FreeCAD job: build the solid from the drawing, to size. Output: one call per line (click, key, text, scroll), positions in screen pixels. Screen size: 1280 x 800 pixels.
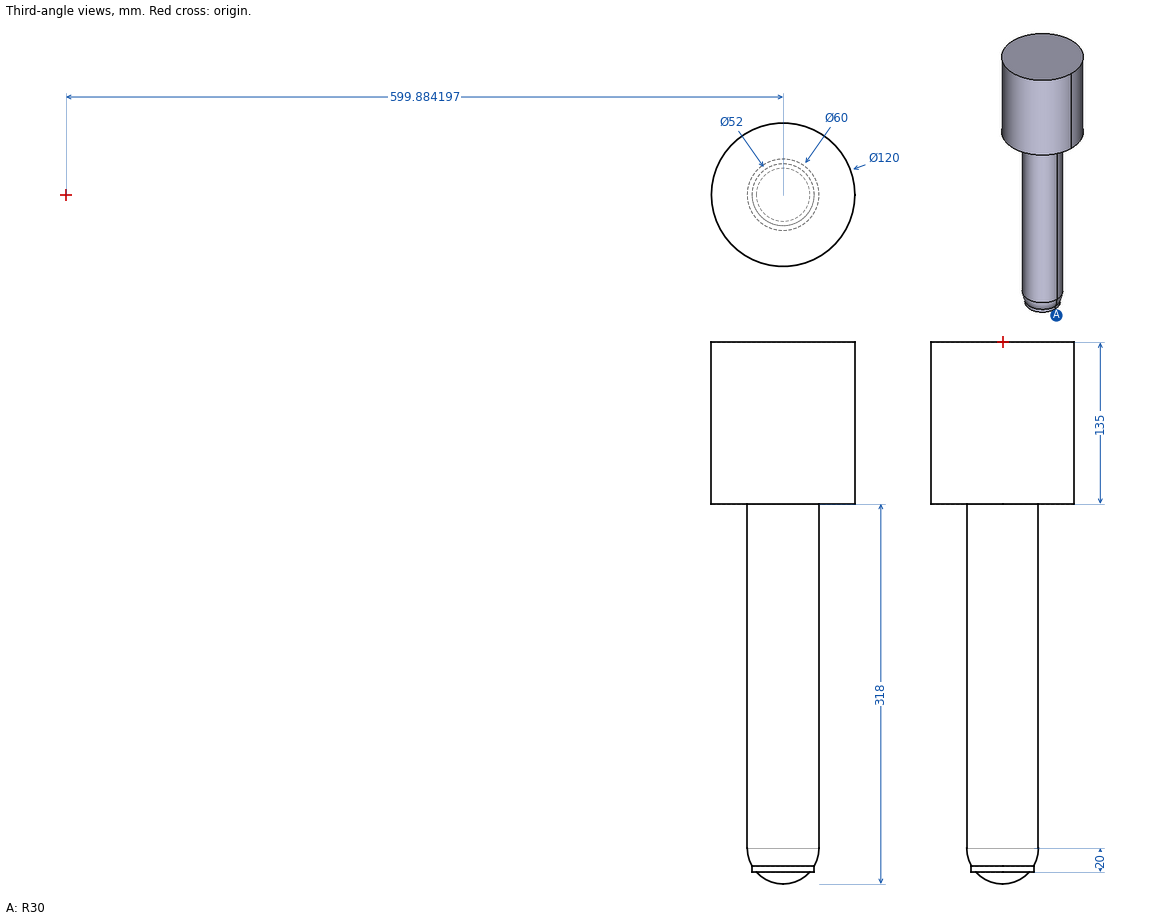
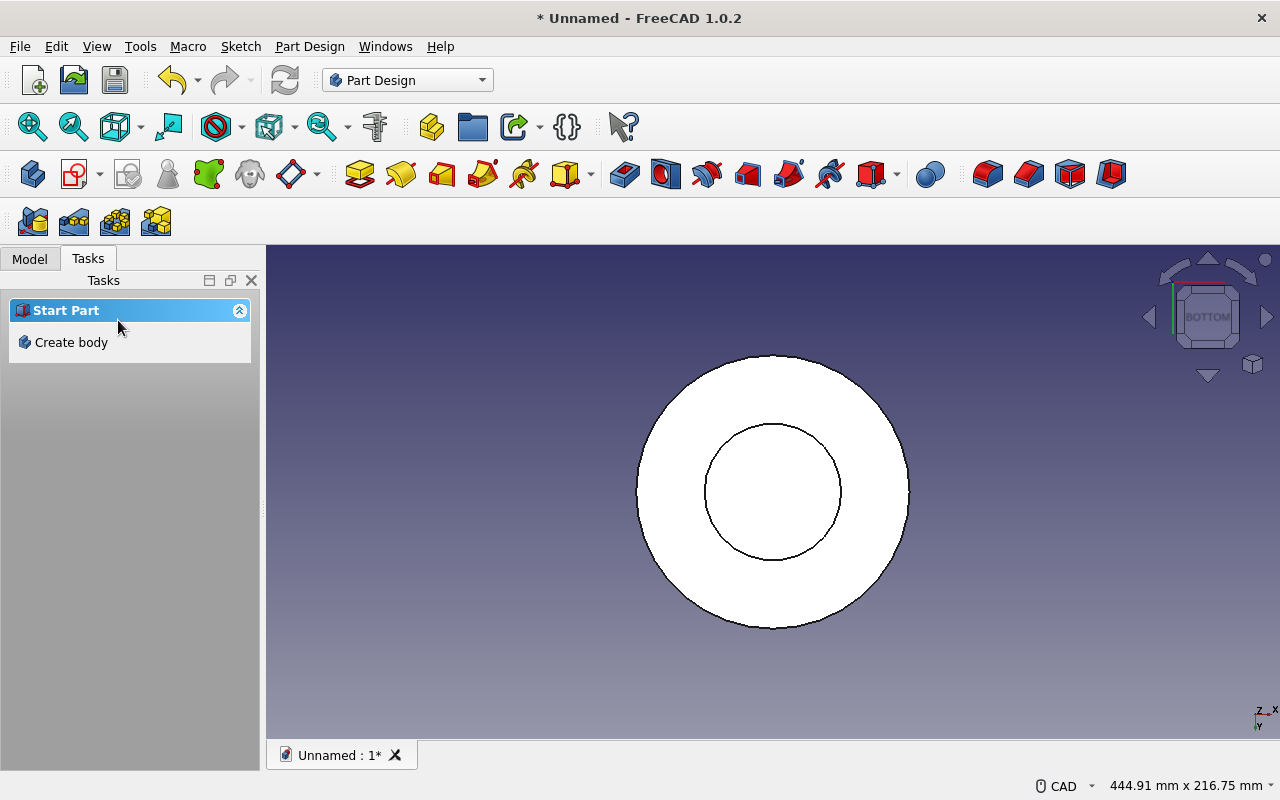
click(704, 491)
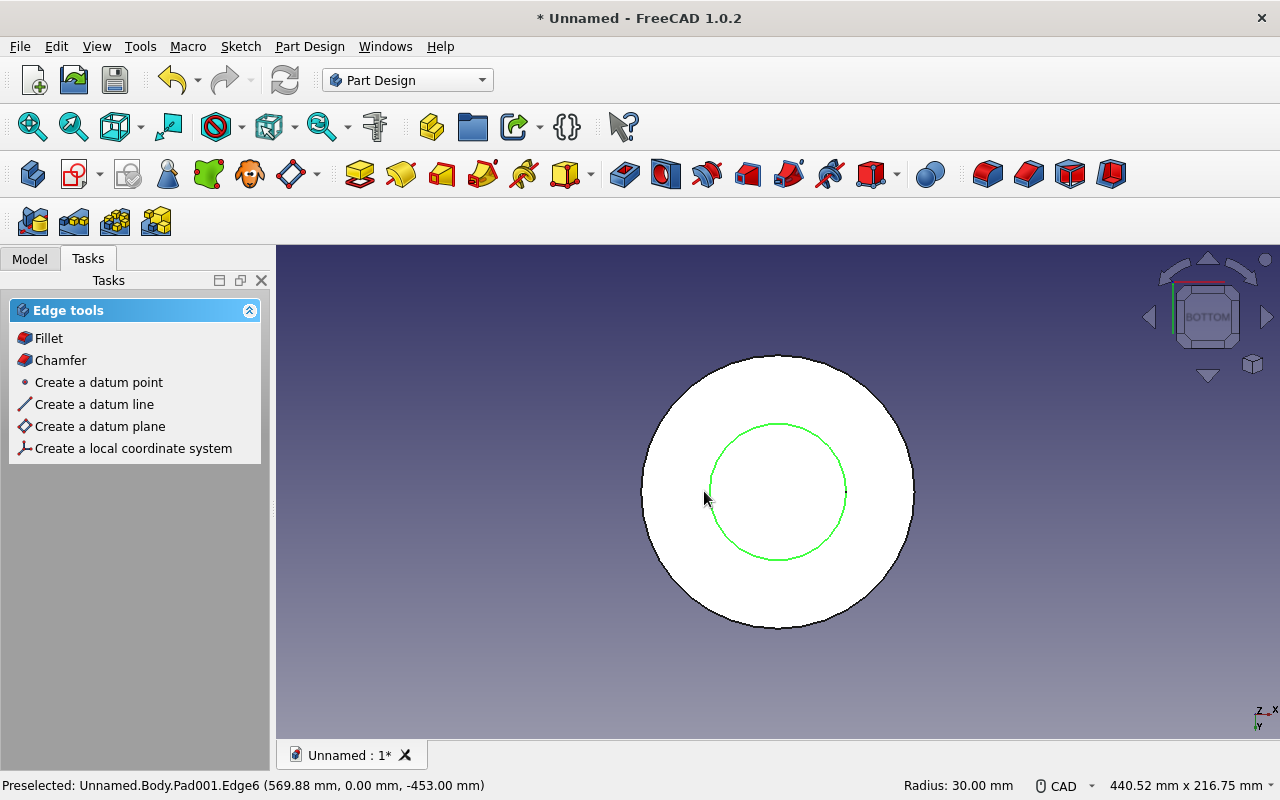
click(988, 174)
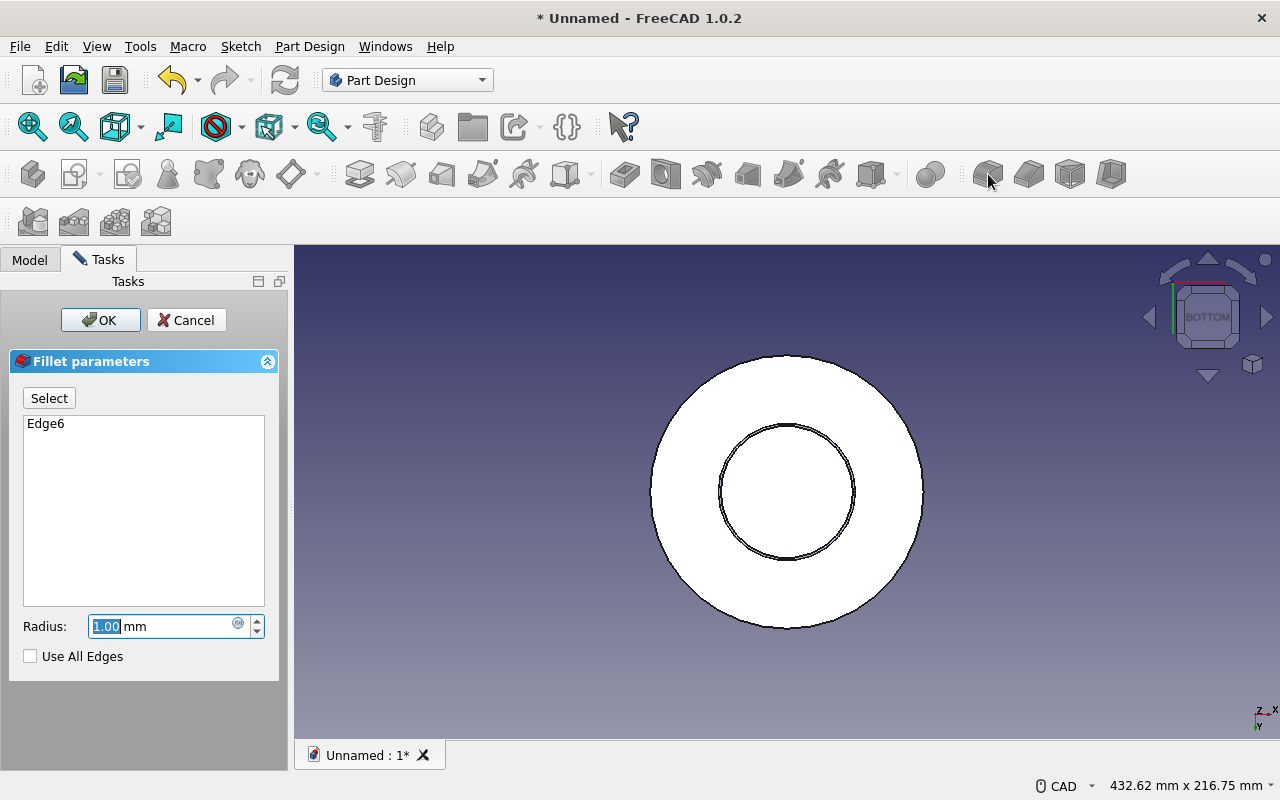
text(30)
key(Tab)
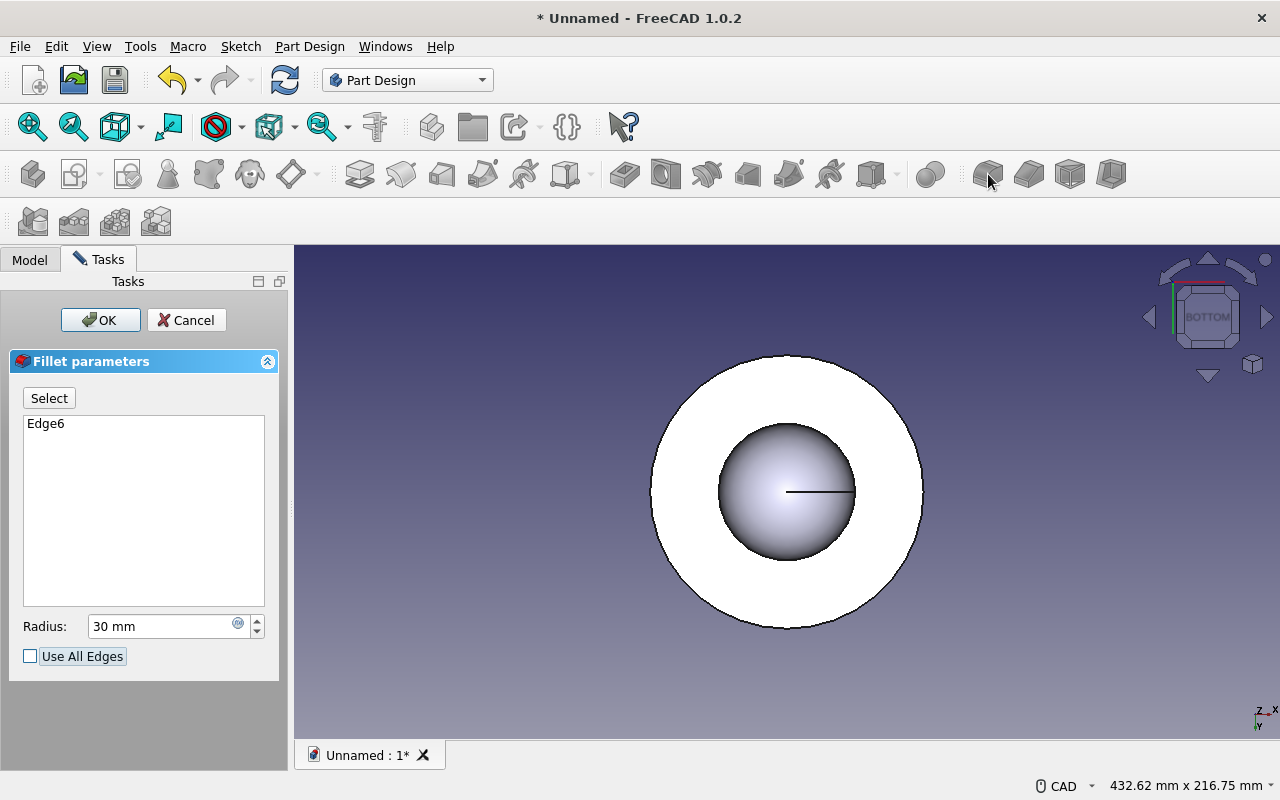
click(101, 320)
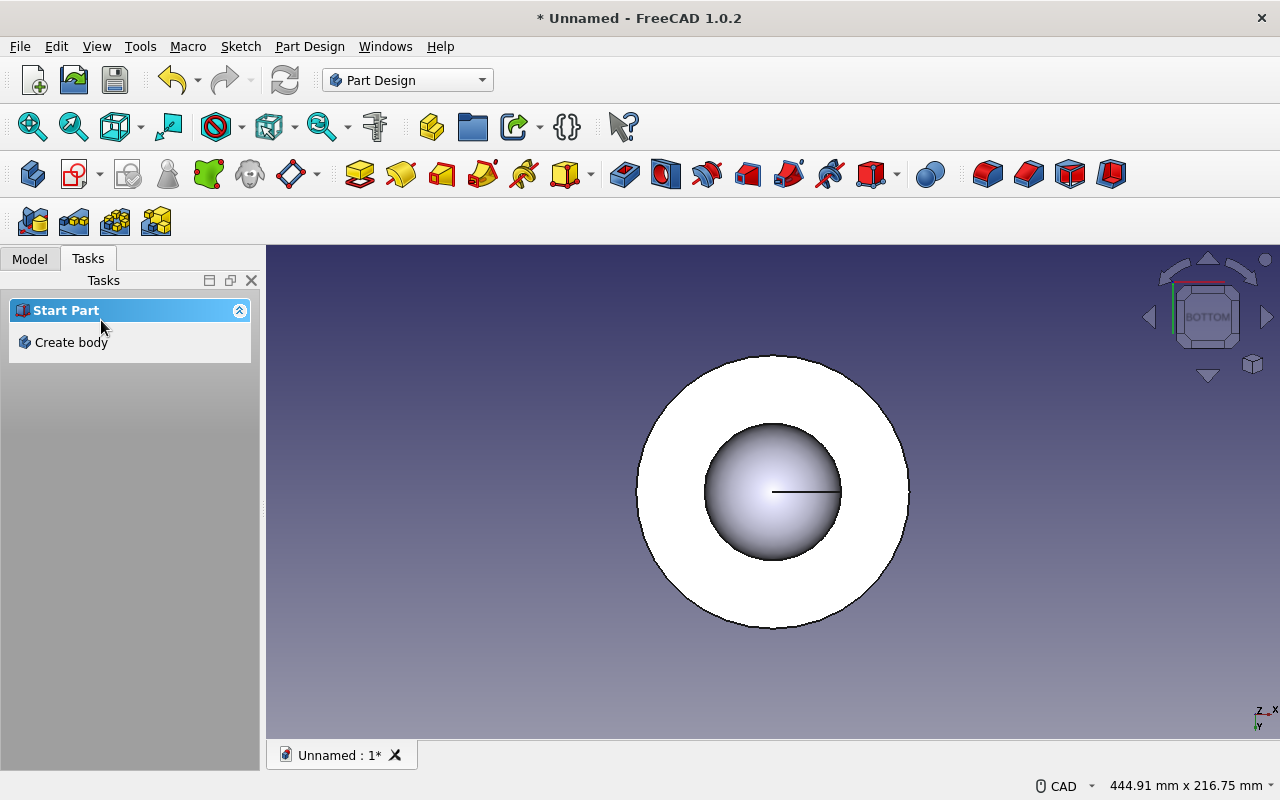
click(30, 258)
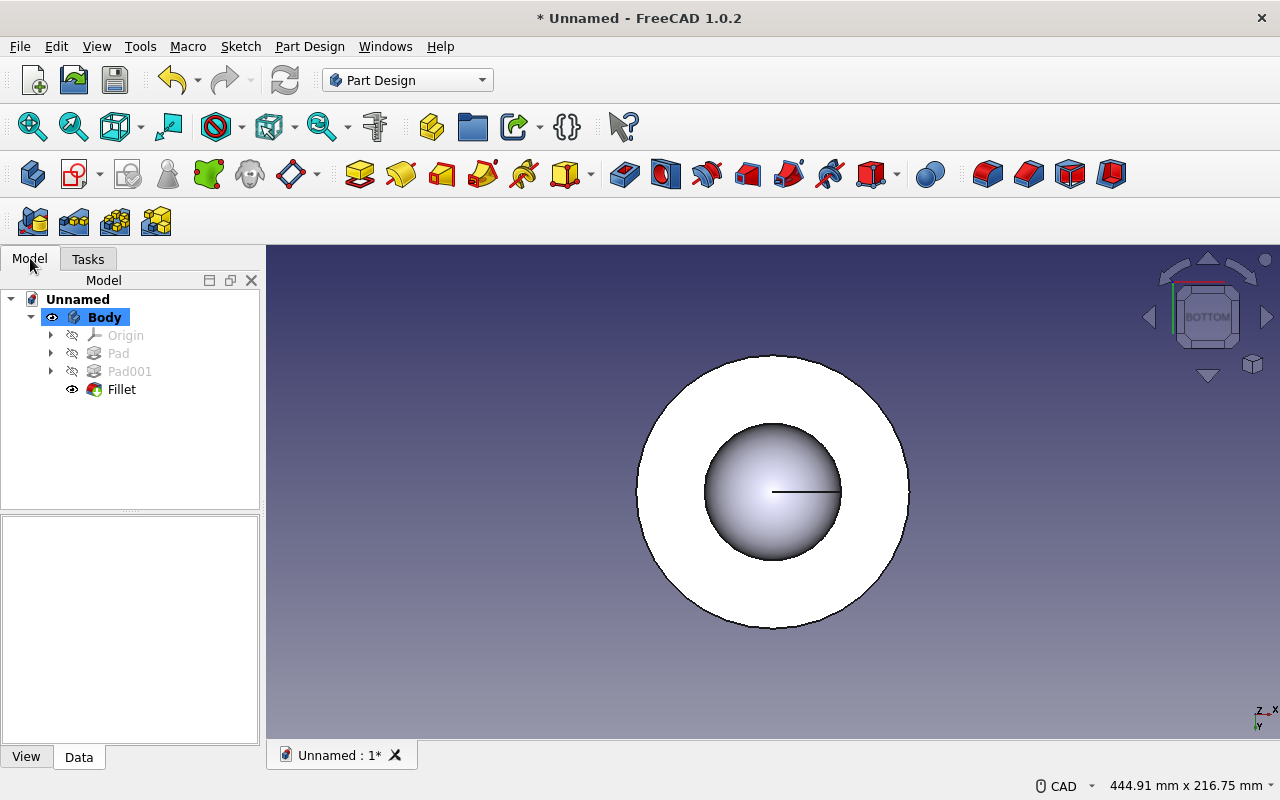
click(51, 335)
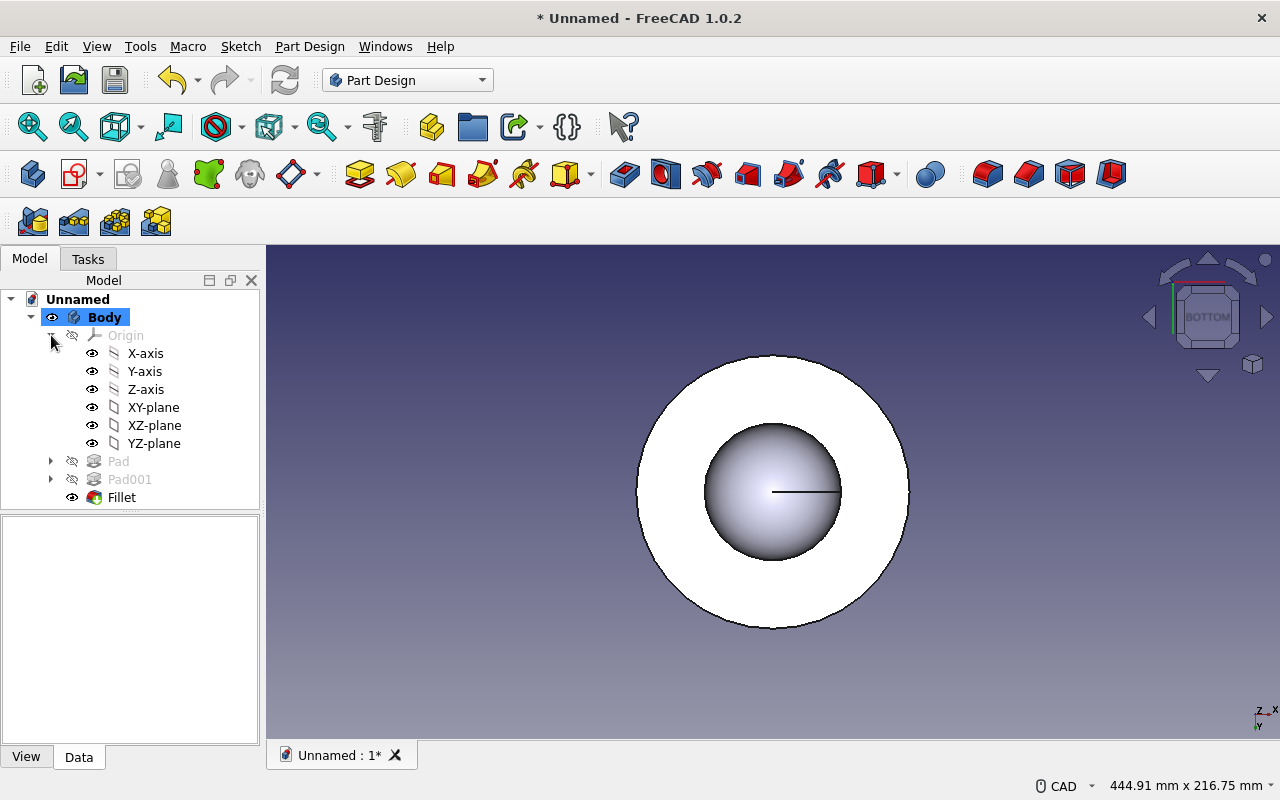
click(137, 407)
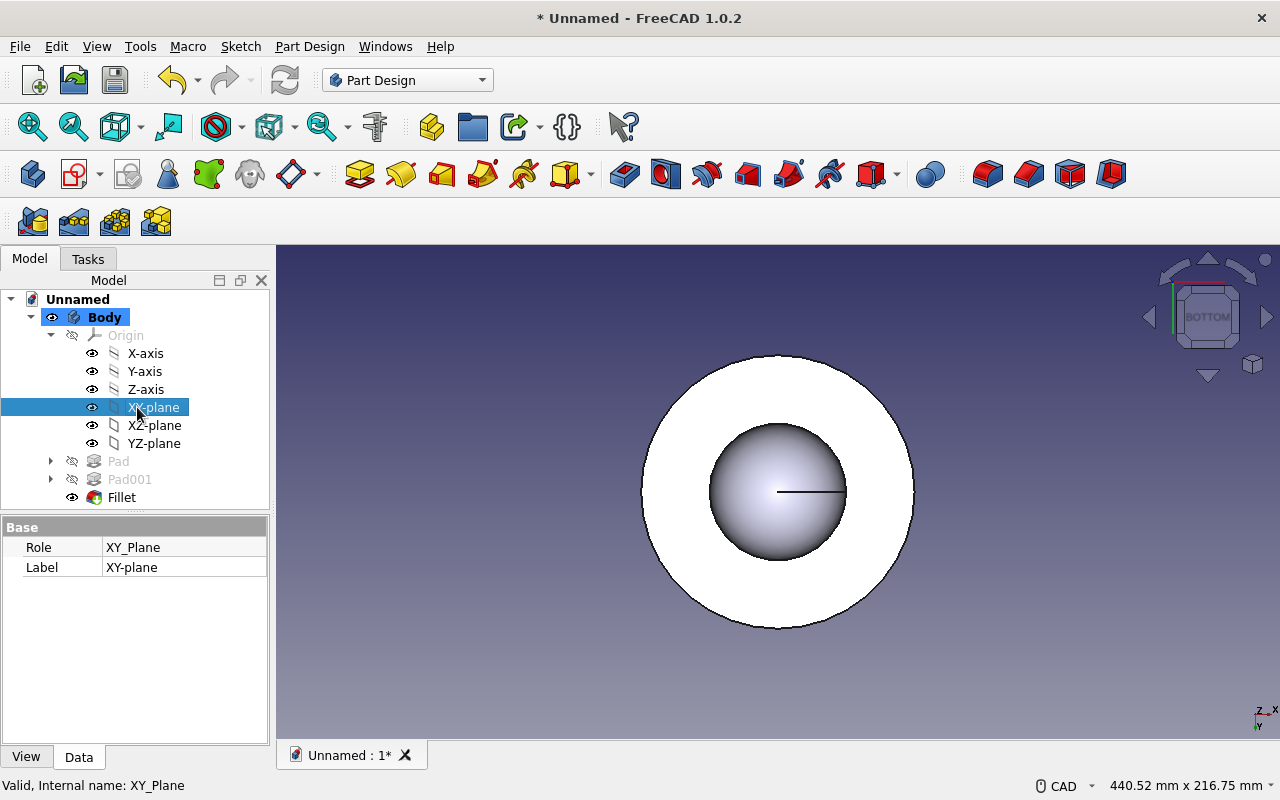
click(290, 174)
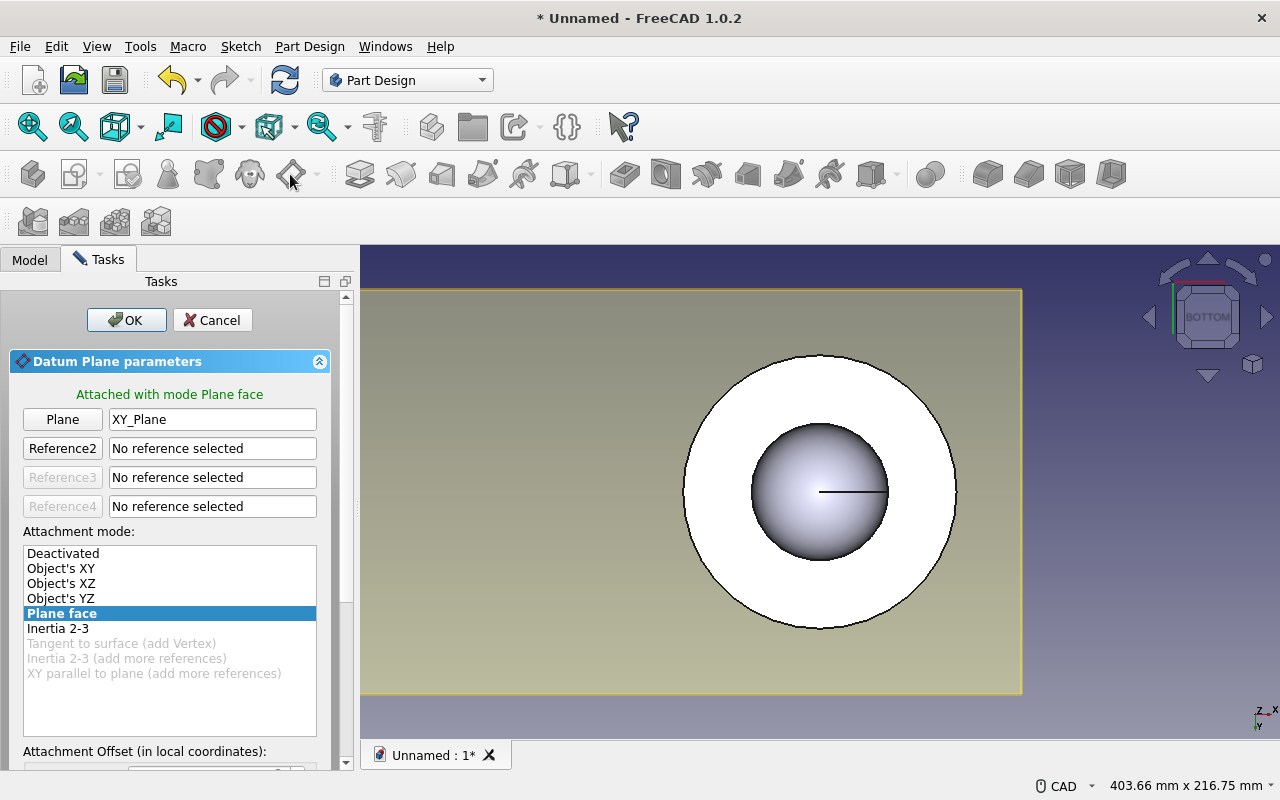
scroll(346, 530, down, 3)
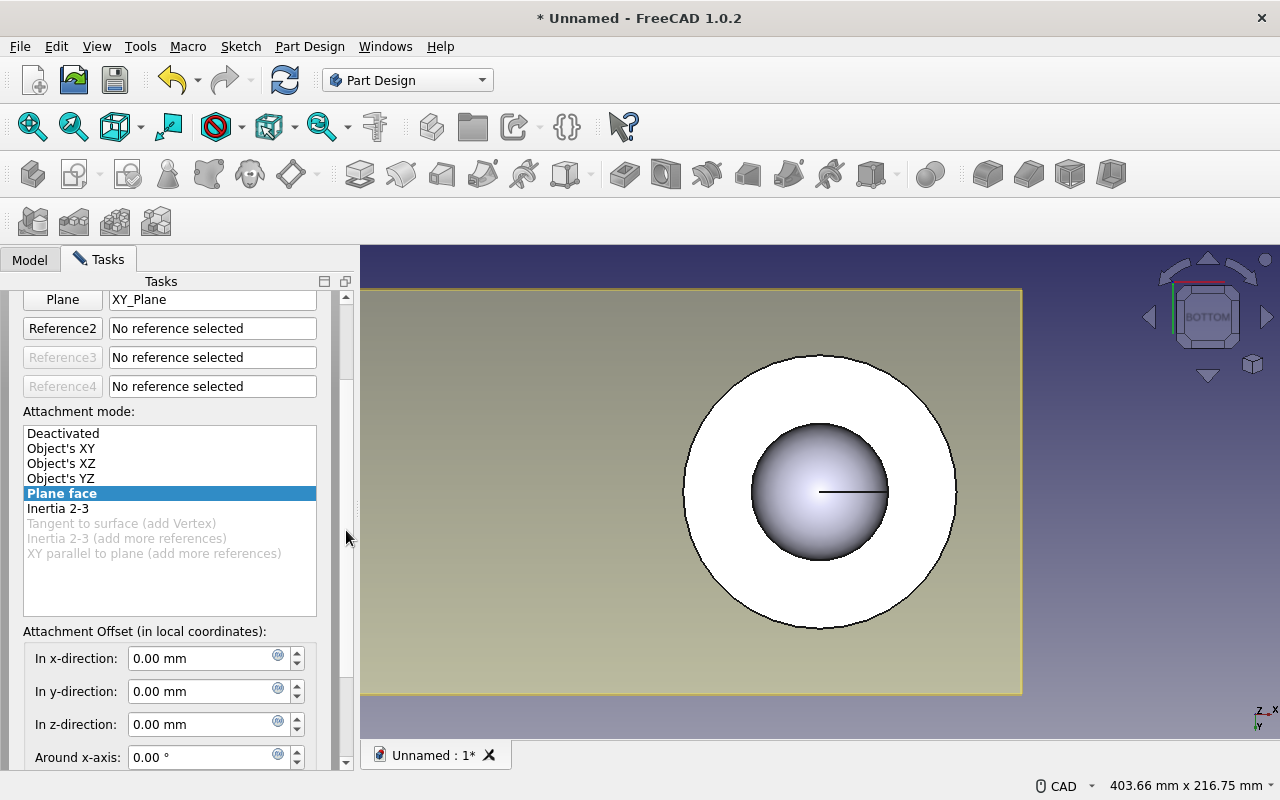
triple_click(210, 664)